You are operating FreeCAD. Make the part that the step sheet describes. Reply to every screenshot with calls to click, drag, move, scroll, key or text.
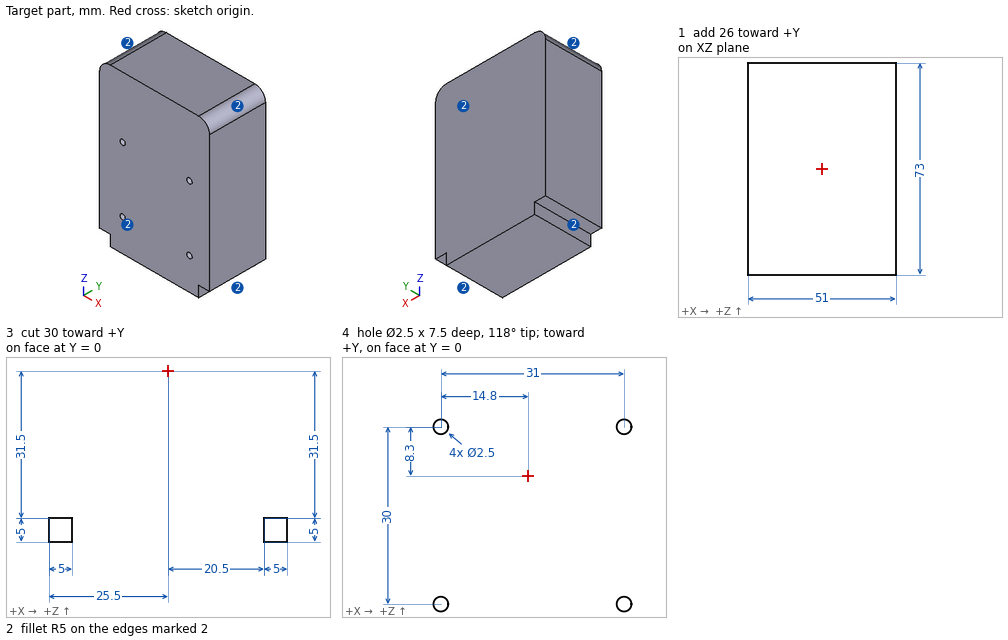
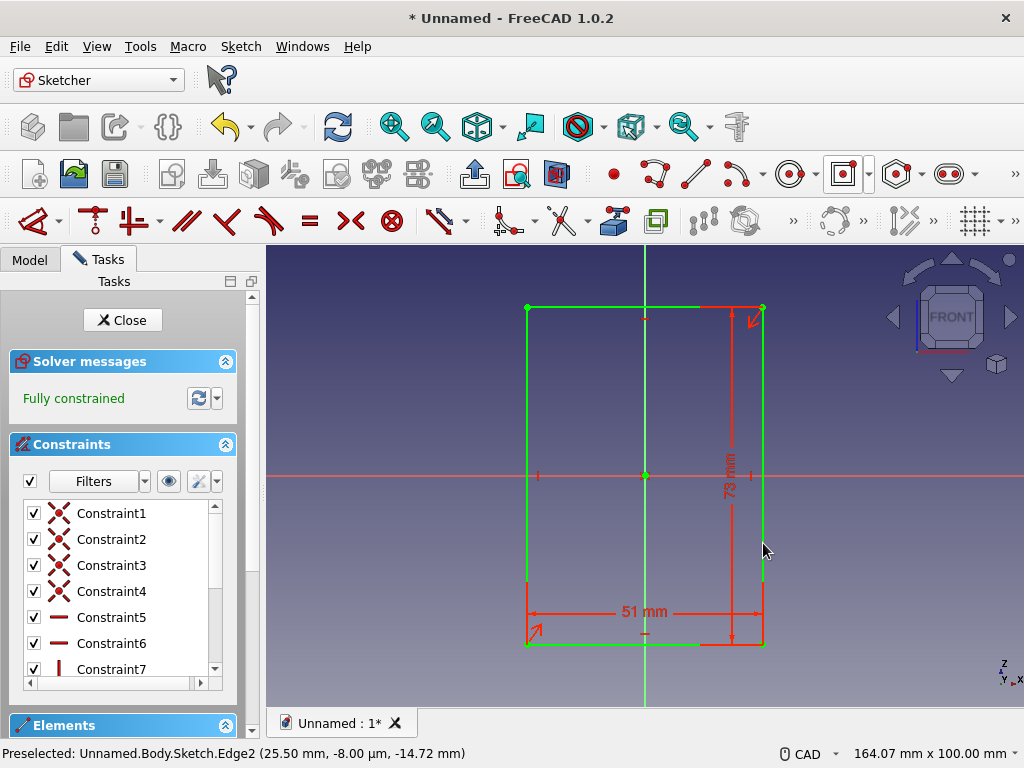
click(123, 320)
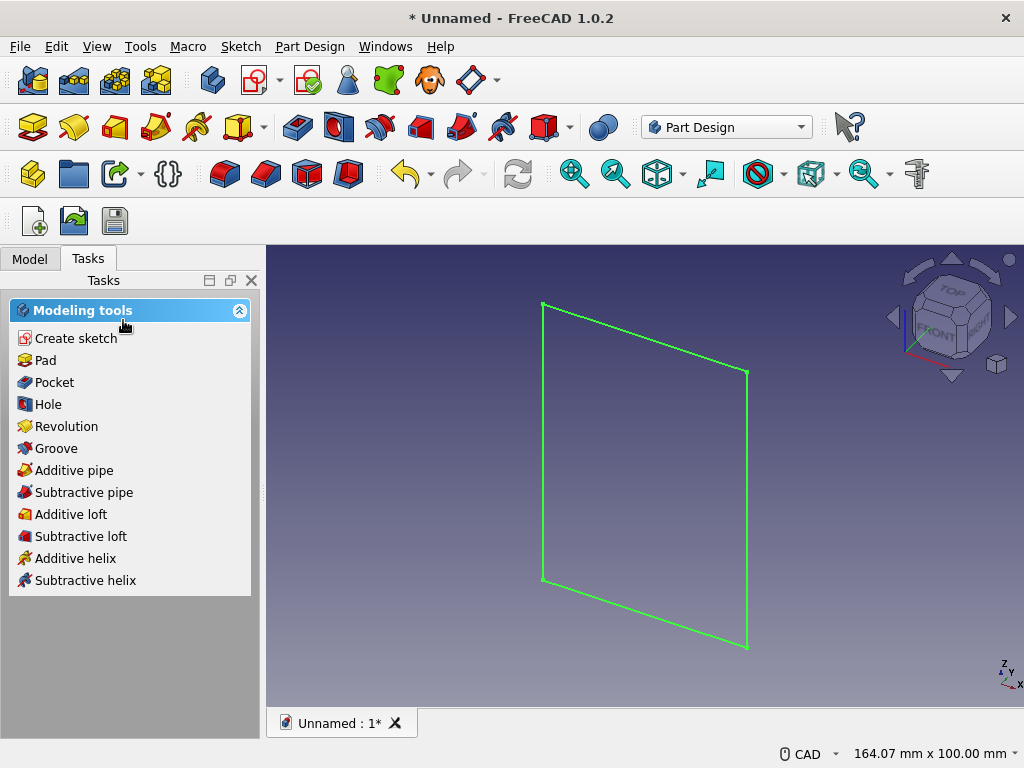
click(33, 128)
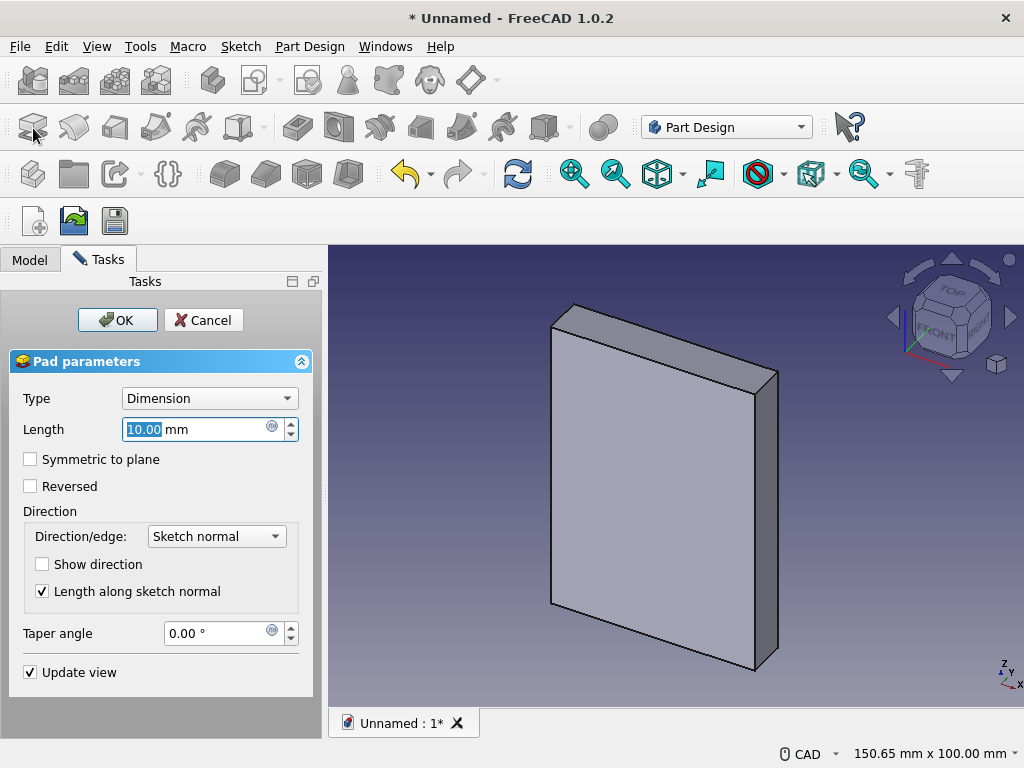
text(26)
key(Tab)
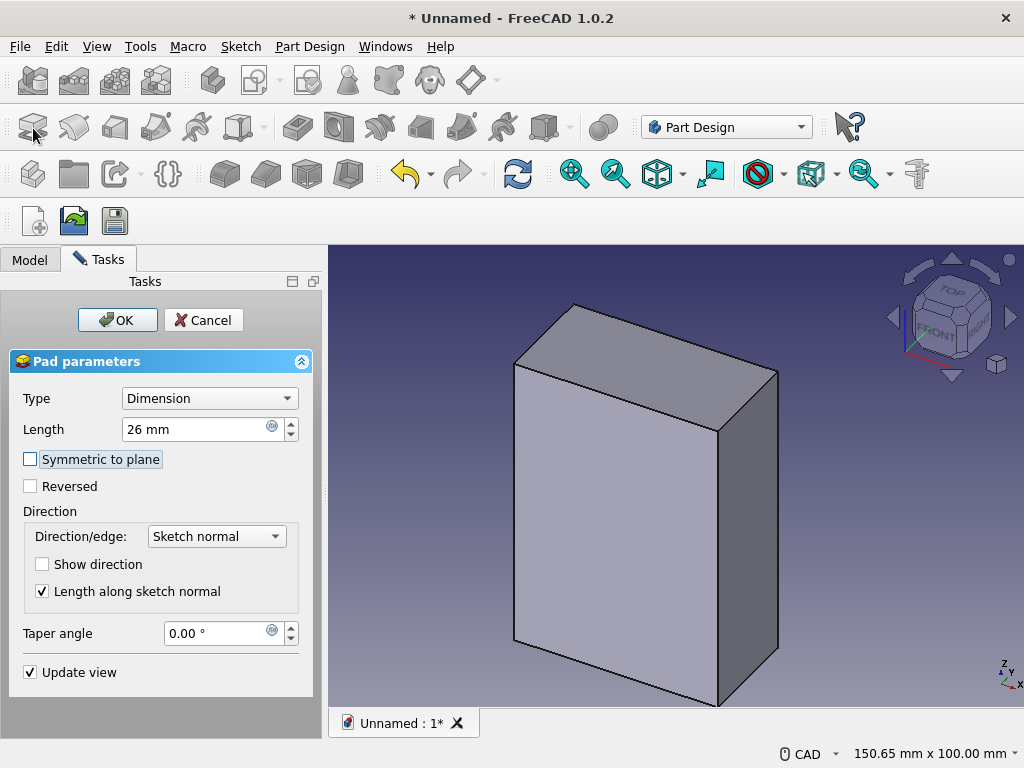
click(31, 486)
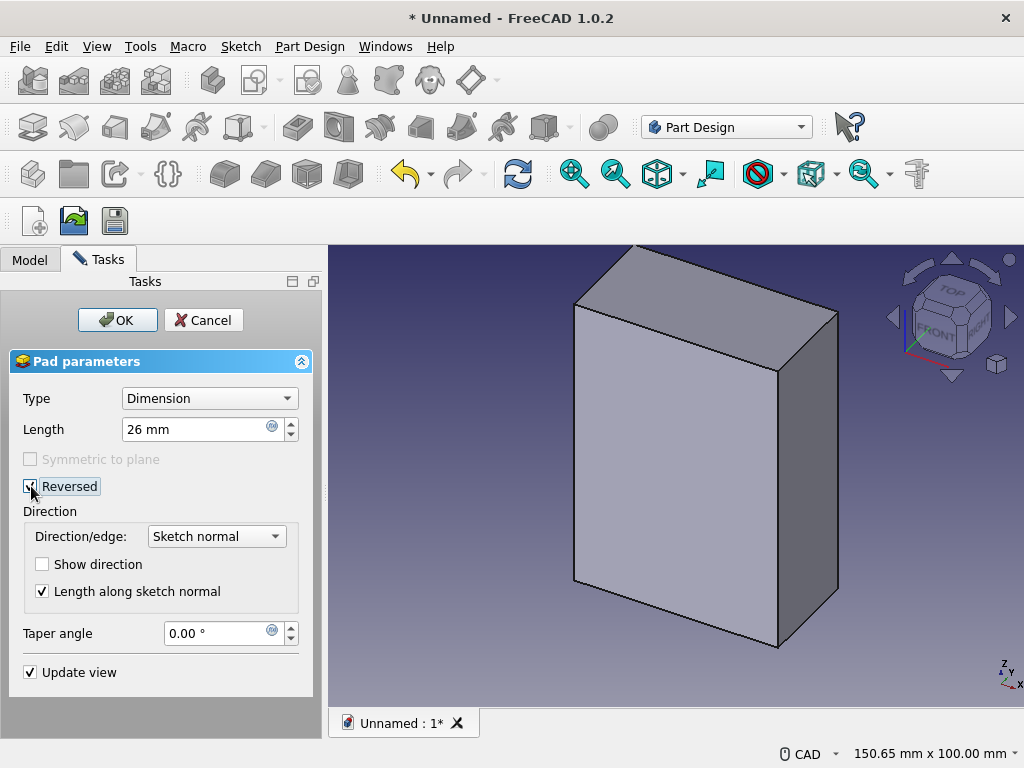
click(118, 320)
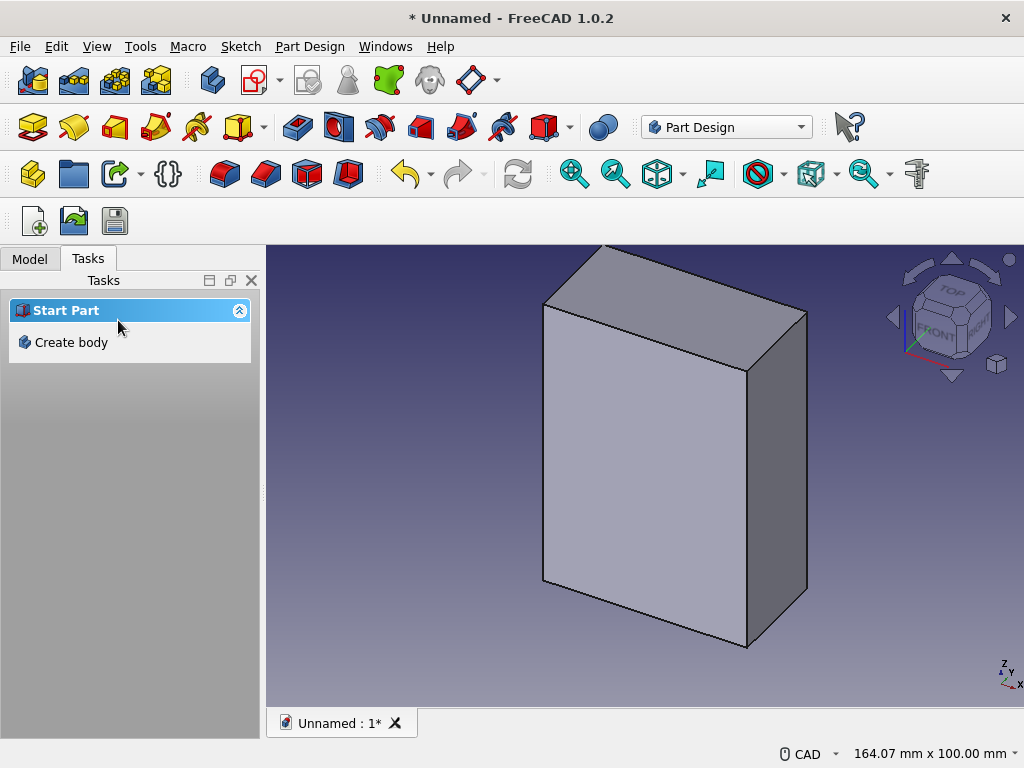
click(575, 174)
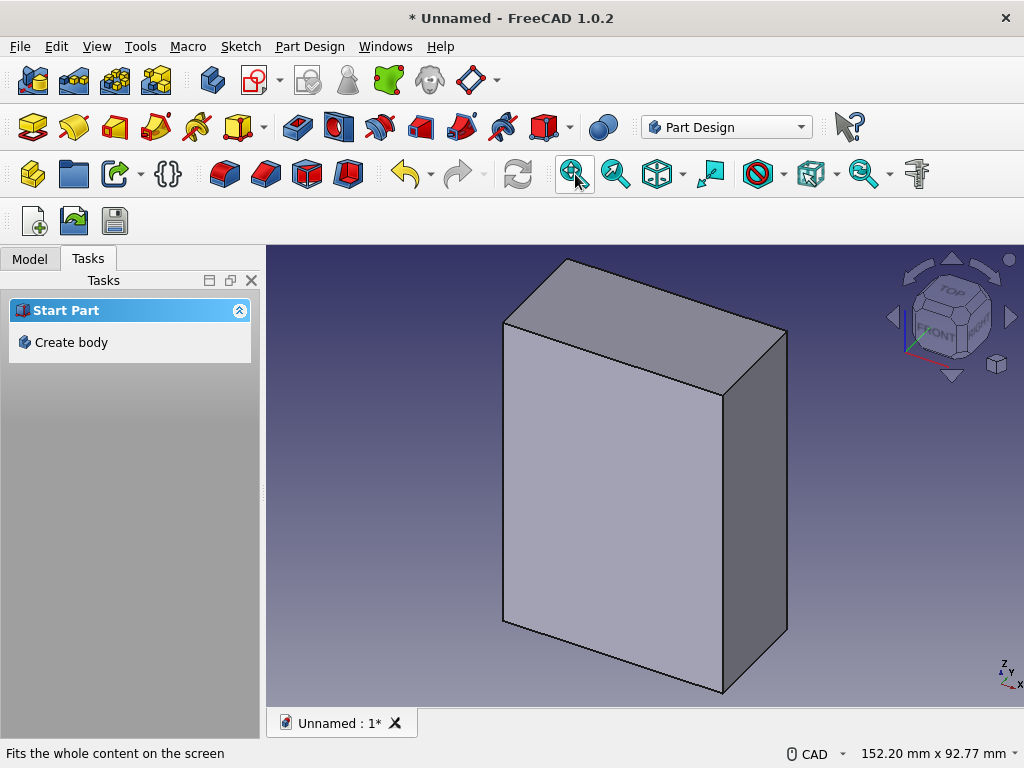
click(755, 363)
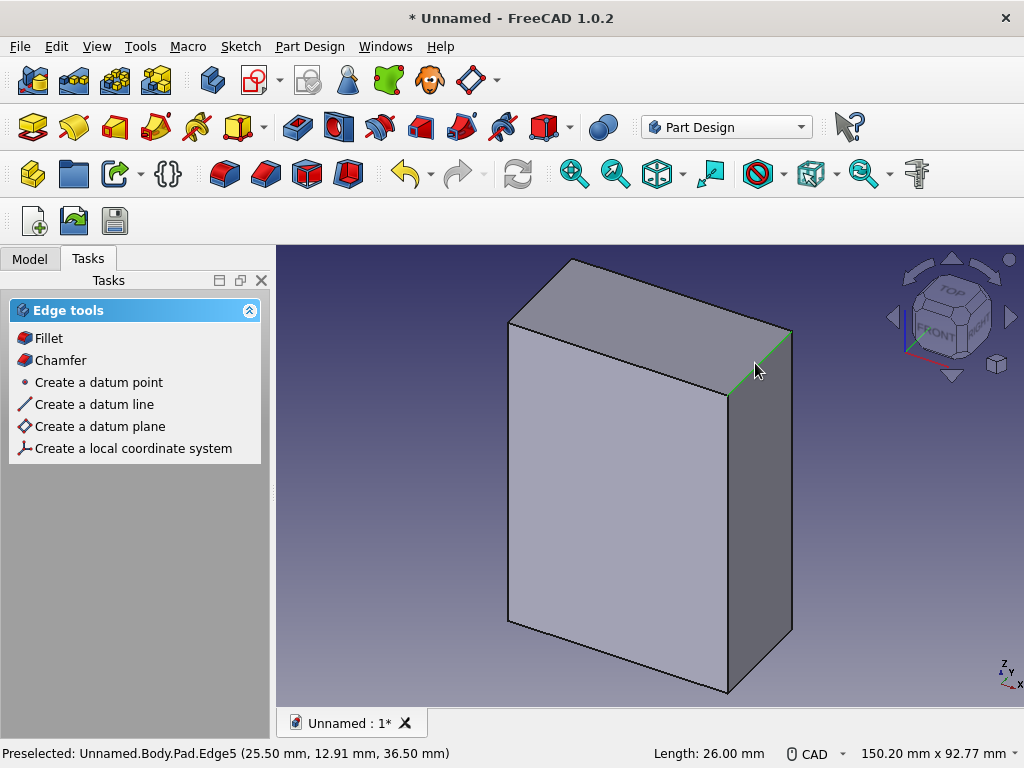
key(0)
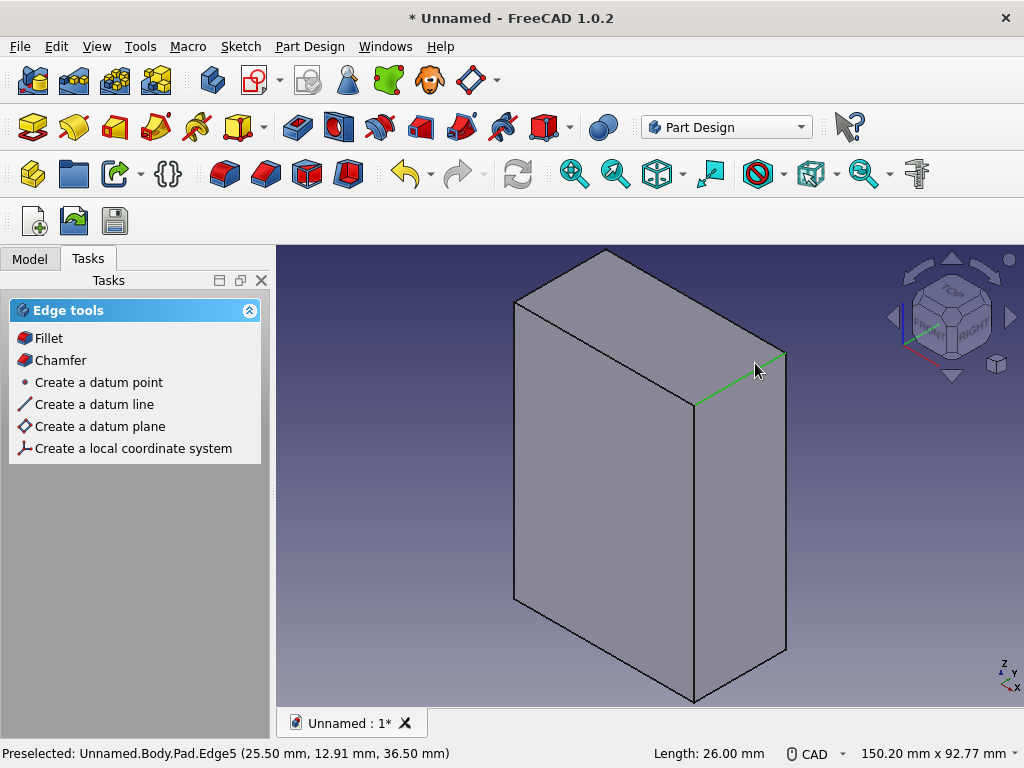
key(2)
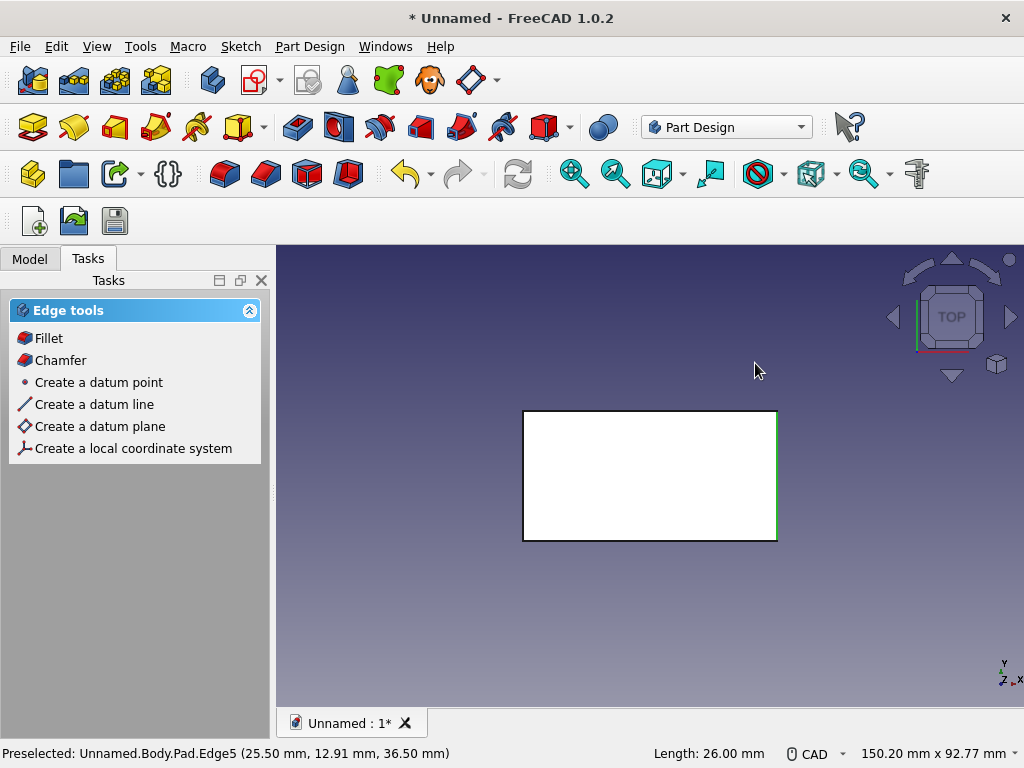
click(575, 174)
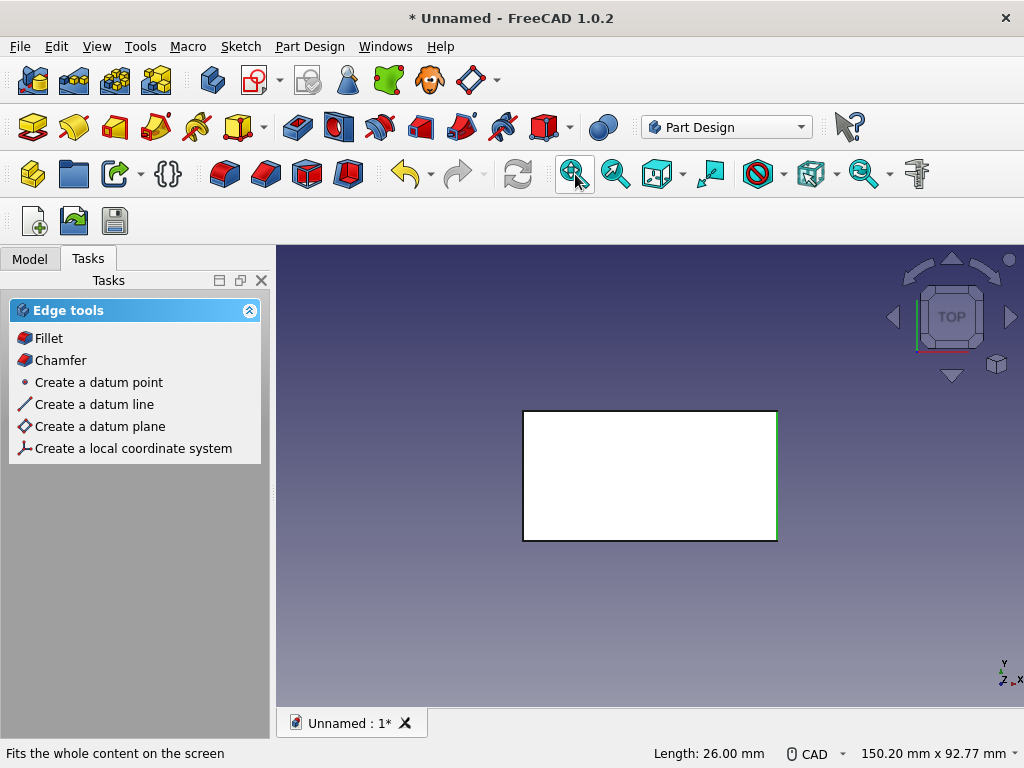
click(523, 475, ctrl)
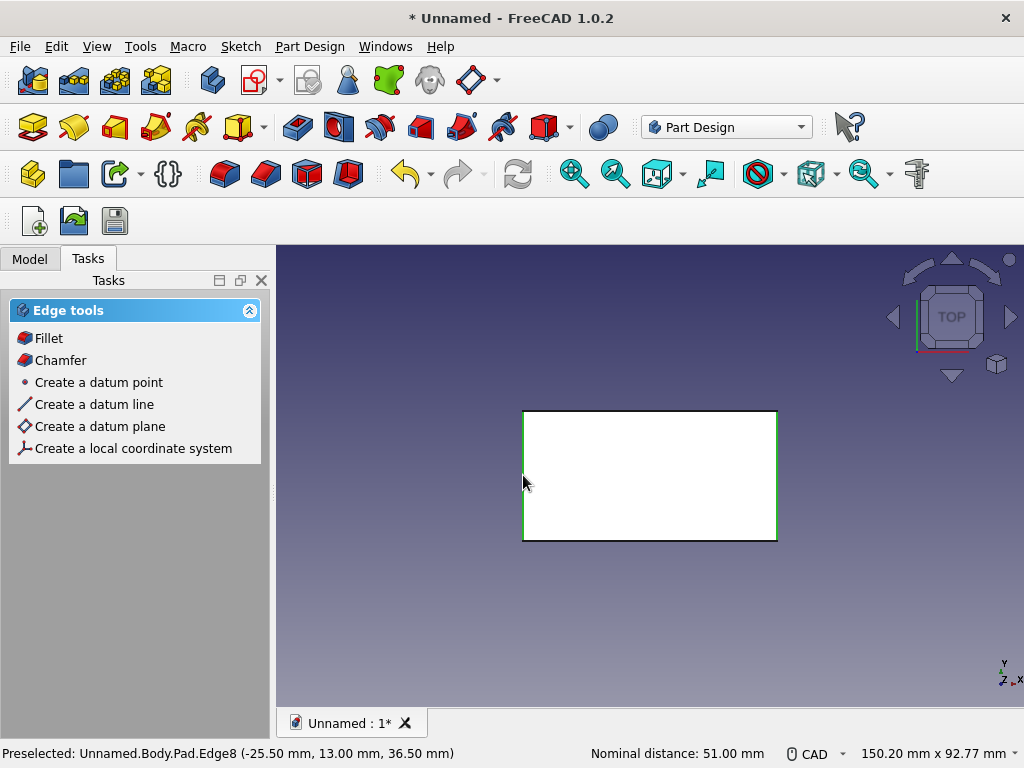
key(1)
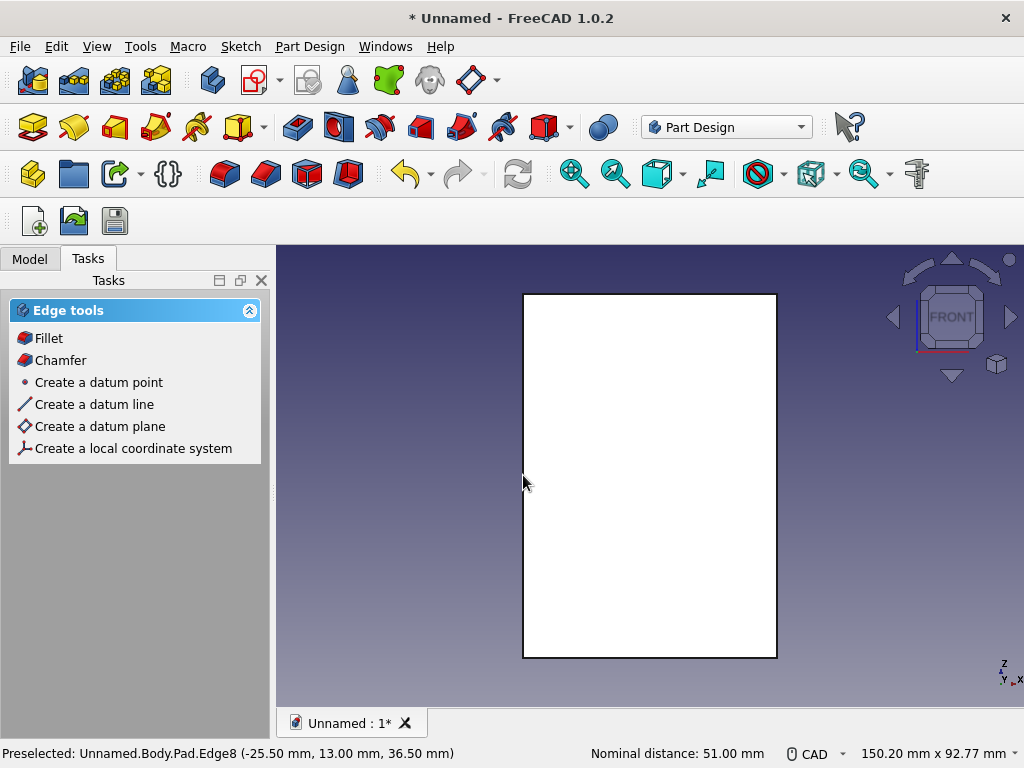
key(3)